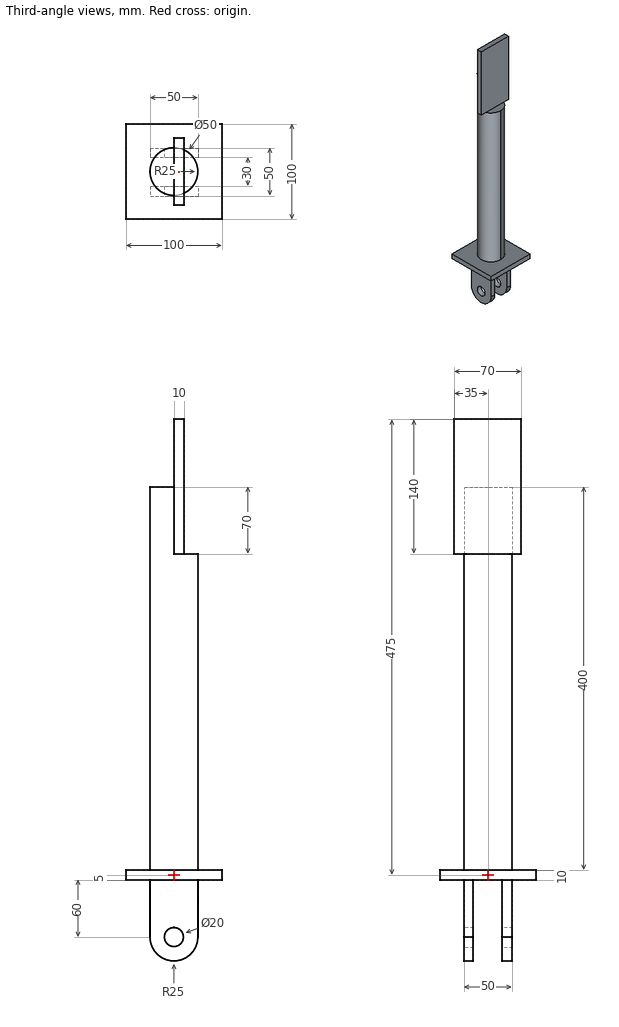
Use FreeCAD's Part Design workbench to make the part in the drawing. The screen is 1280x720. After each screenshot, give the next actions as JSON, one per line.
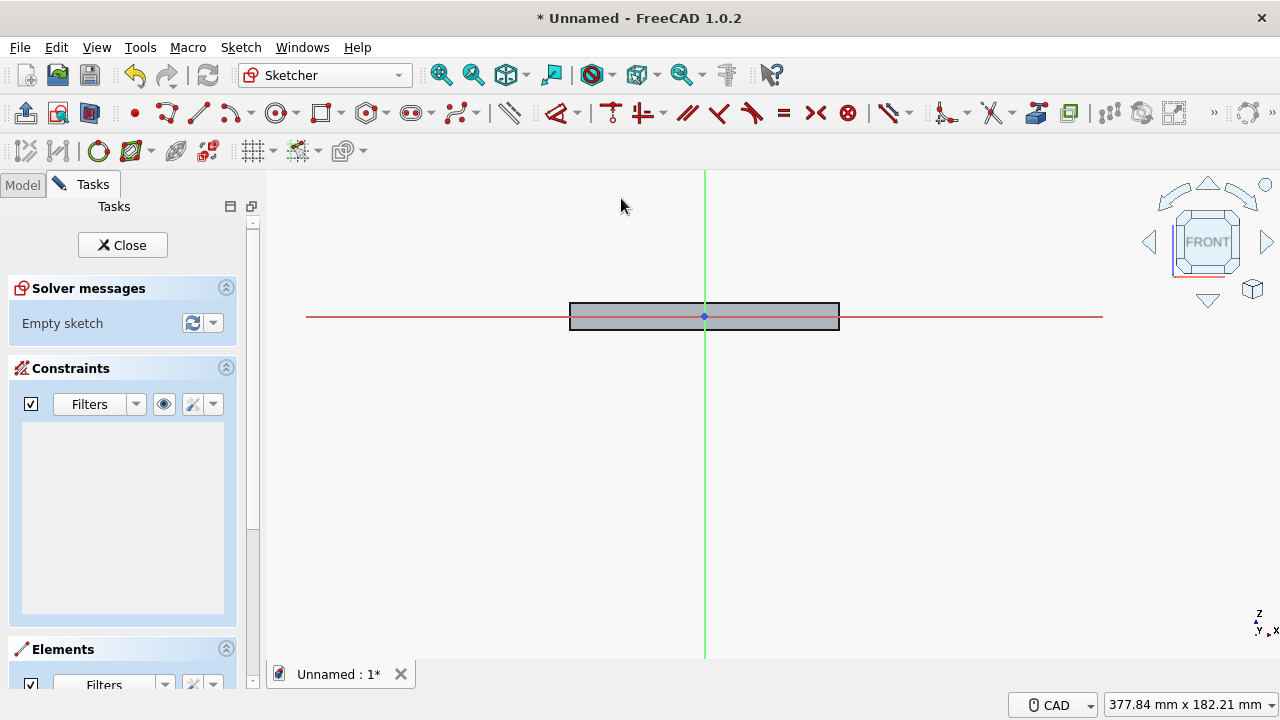
{"action": "key", "text": "g m"}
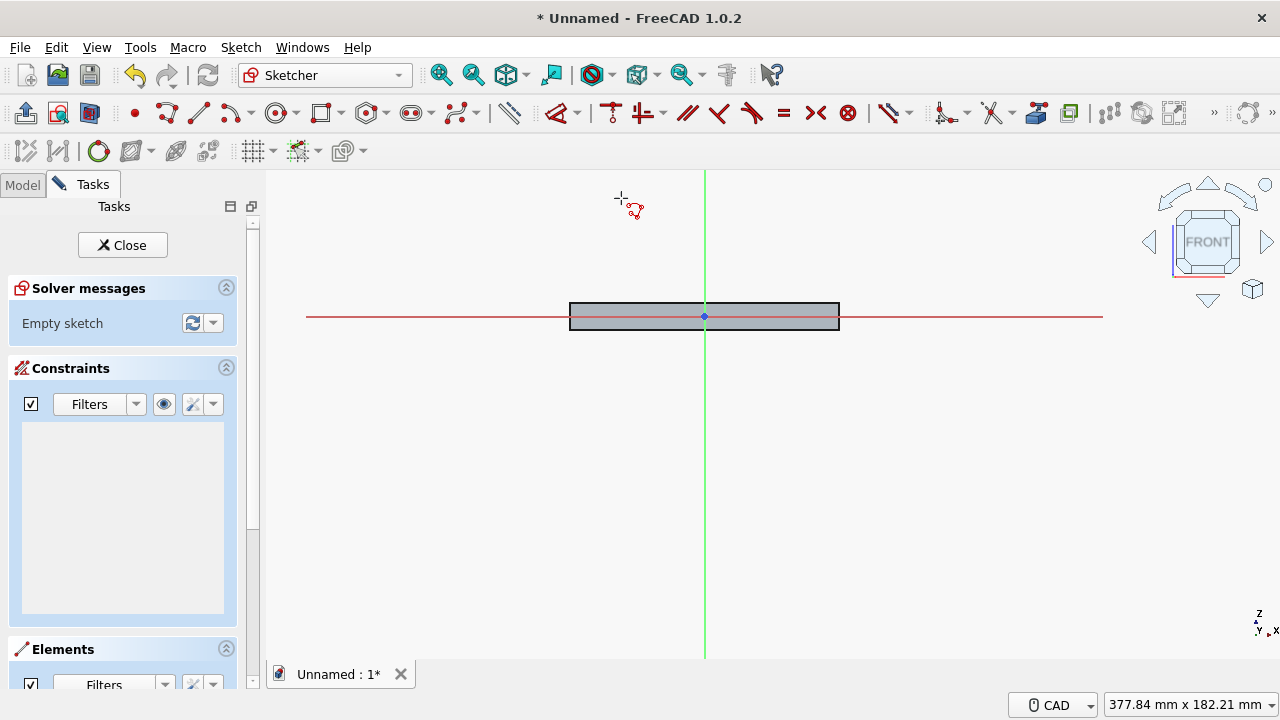
{"action": "left_click", "coordinate": [637, 491]}
{"action": "left_click", "coordinate": [637, 330]}
{"action": "left_click", "coordinate": [772, 330]}
{"action": "left_click", "coordinate": [772, 491]}
{"action": "right_click", "coordinate": [772, 491]}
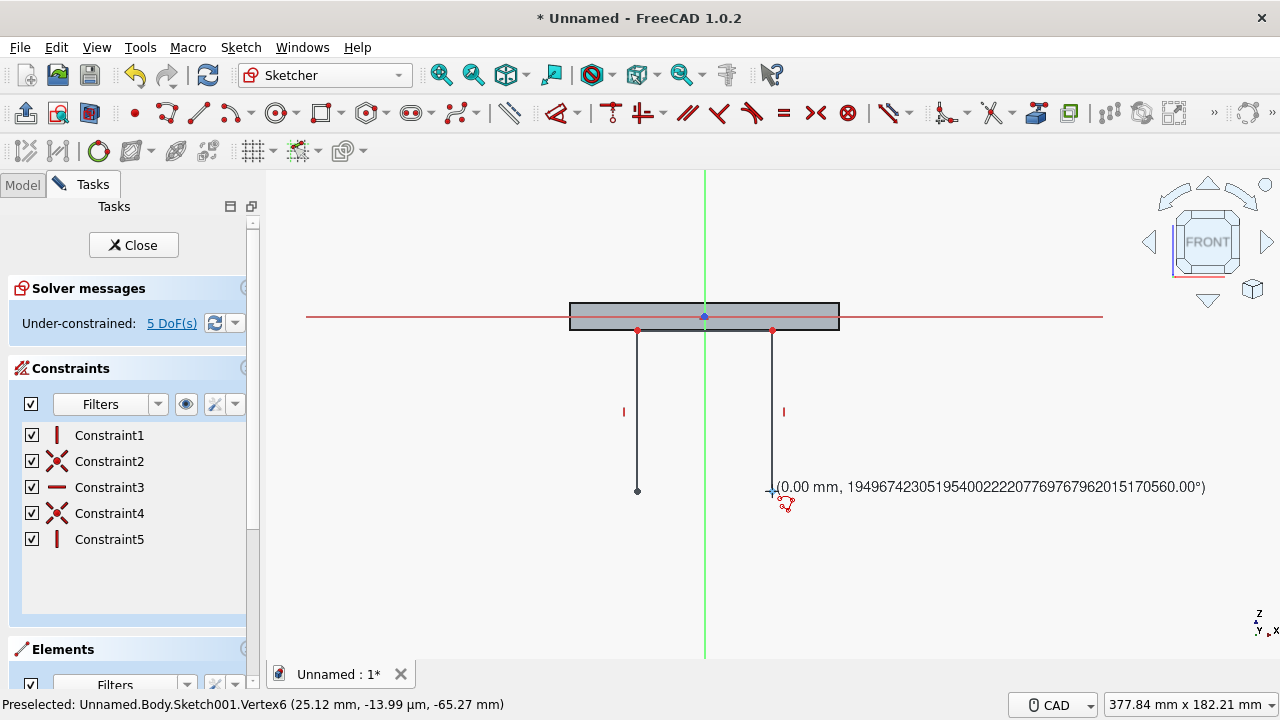
{"action": "key", "text": "g 3 a"}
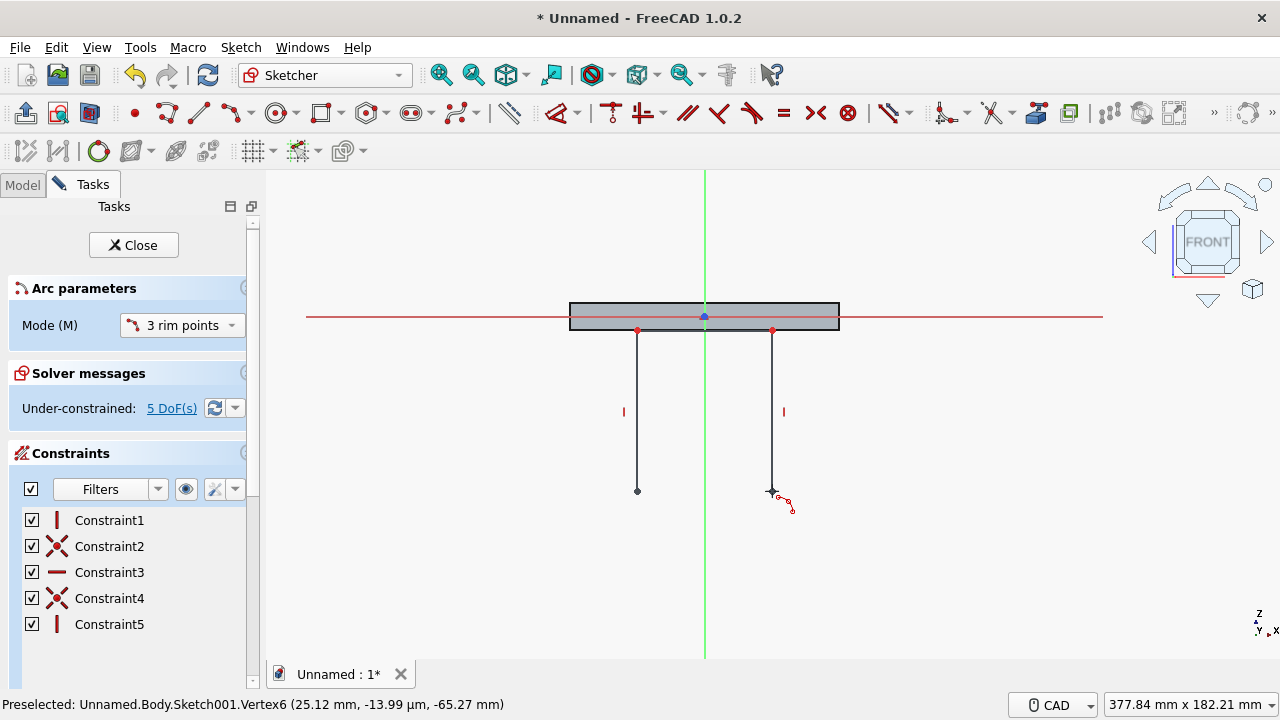
{"action": "left_click", "coordinate": [772, 492]}
{"action": "left_click", "coordinate": [637, 492]}
{"action": "left_click", "coordinate": [684, 555]}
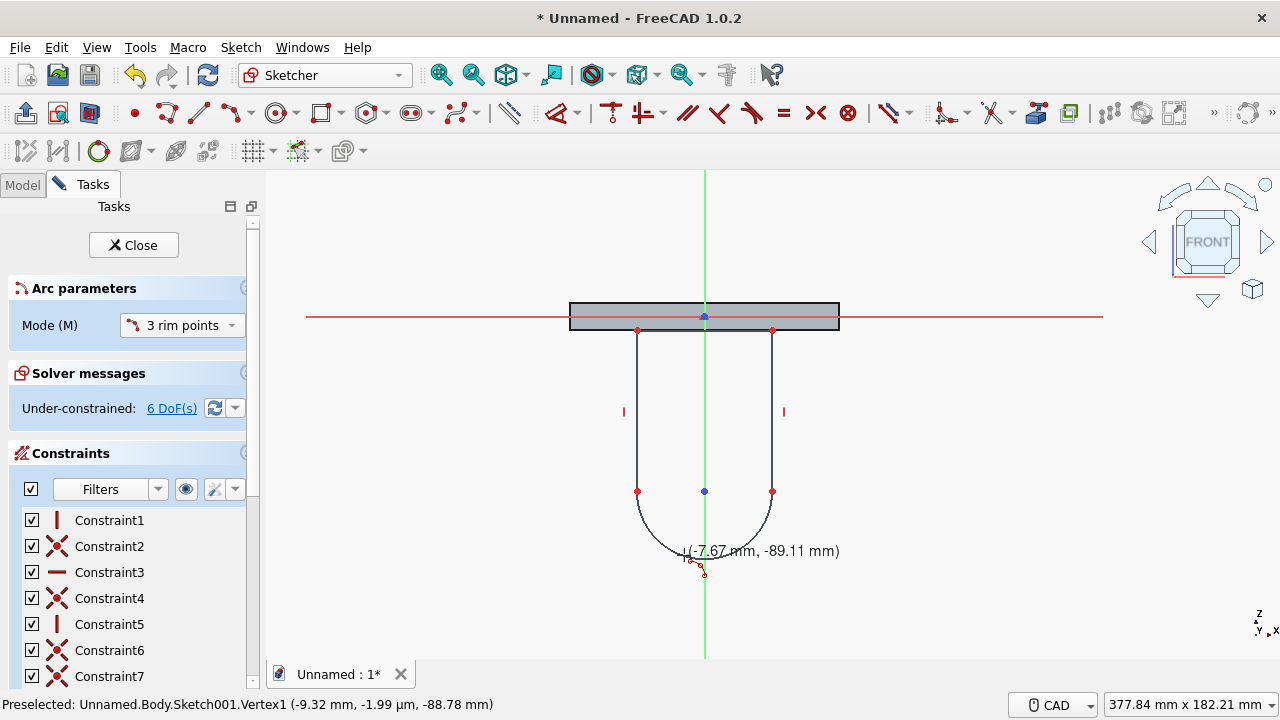
{"action": "key", "text": "g c"}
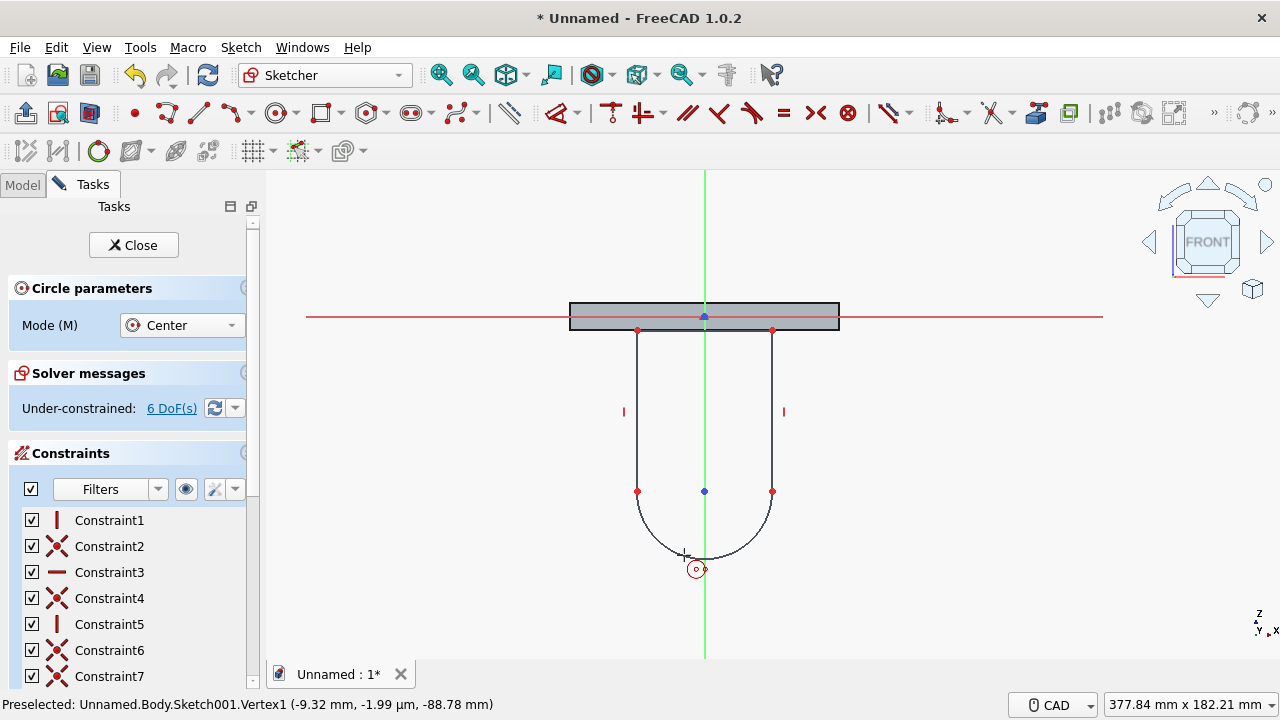
{"action": "left_click", "coordinate": [705, 491]}
{"action": "left_click", "coordinate": [724, 472]}
{"action": "key", "text": "Escape"}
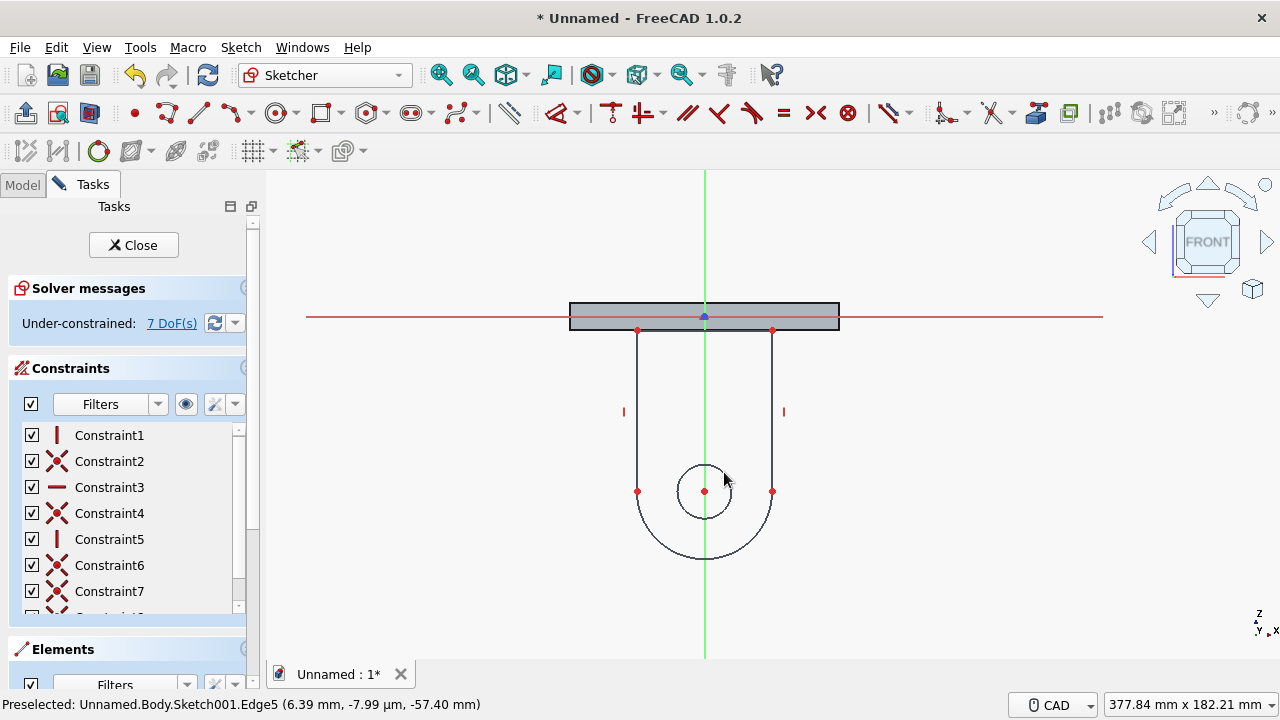
{"action": "left_click", "coordinate": [637, 444]}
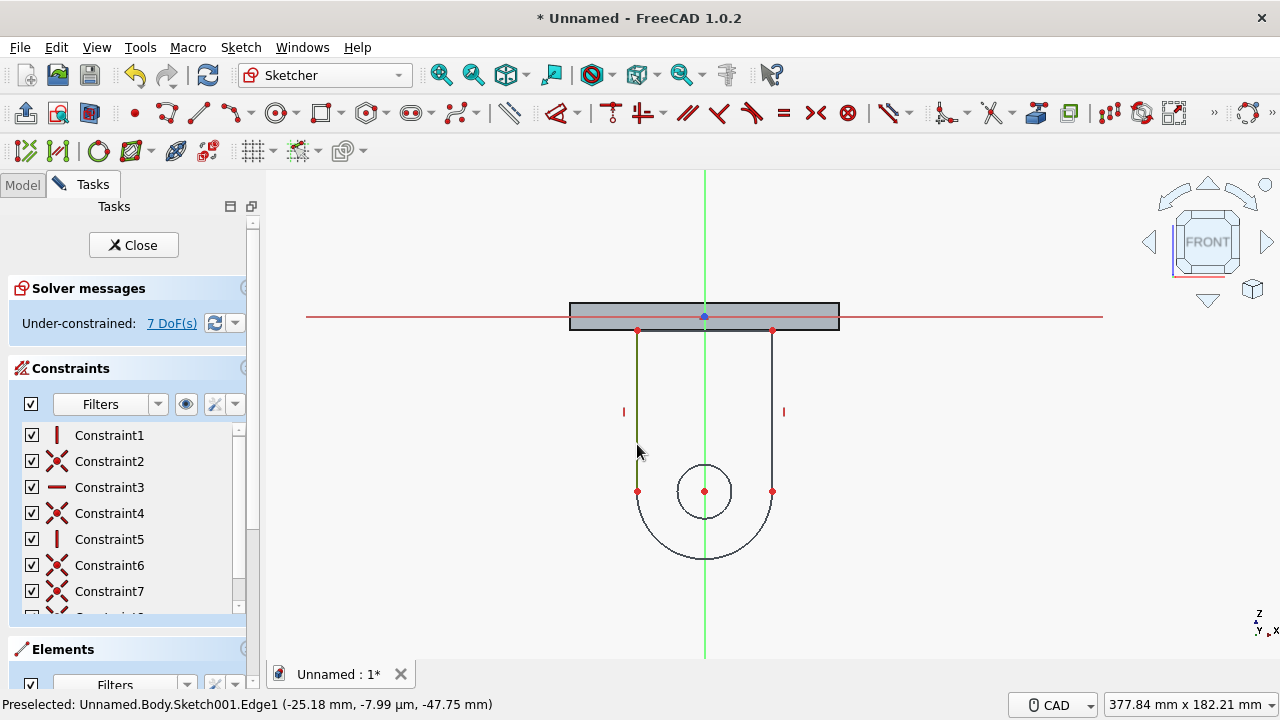
{"action": "left_click", "coordinate": [665, 546]}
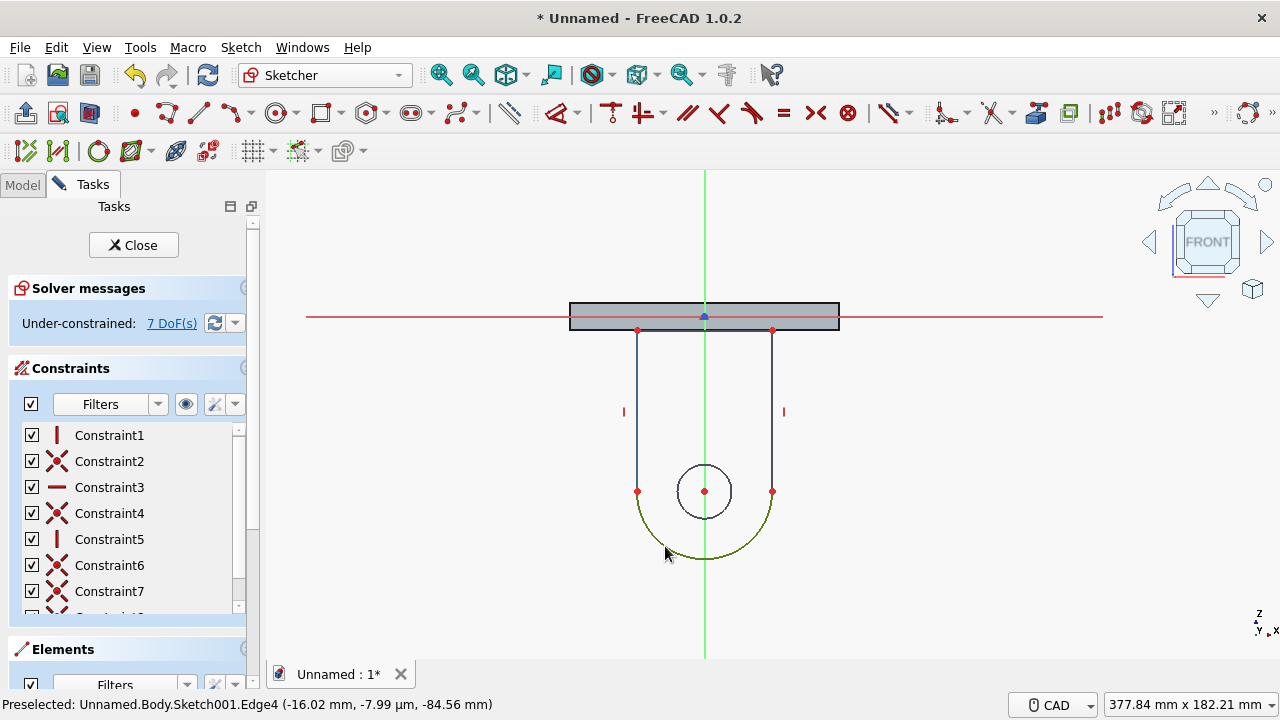
{"action": "key", "text": "t"}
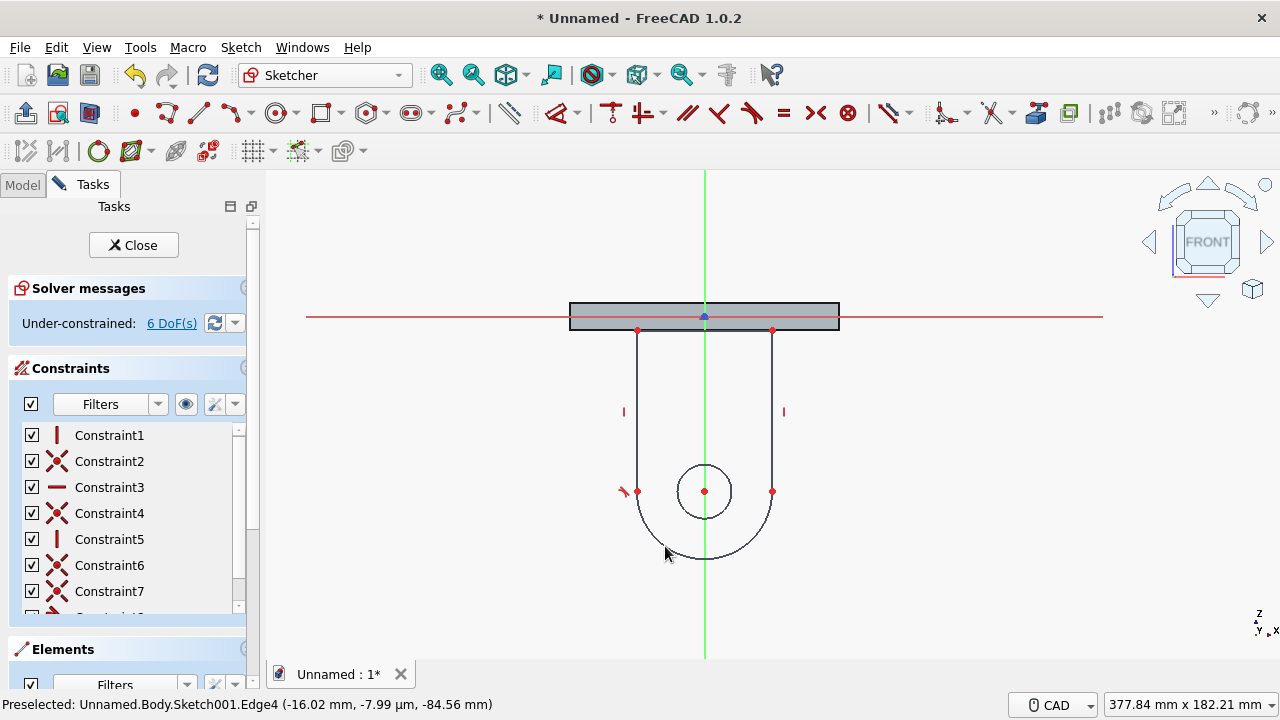
{"action": "left_click", "coordinate": [772, 379]}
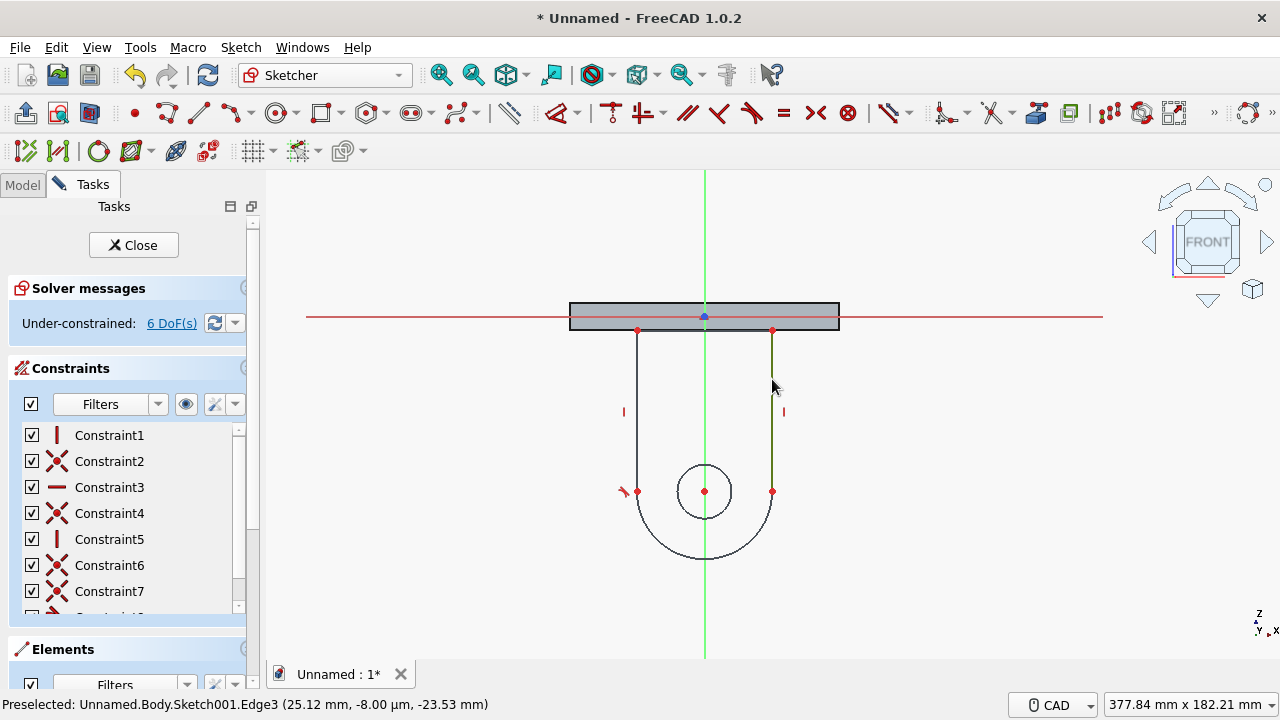
{"action": "left_click", "coordinate": [665, 546]}